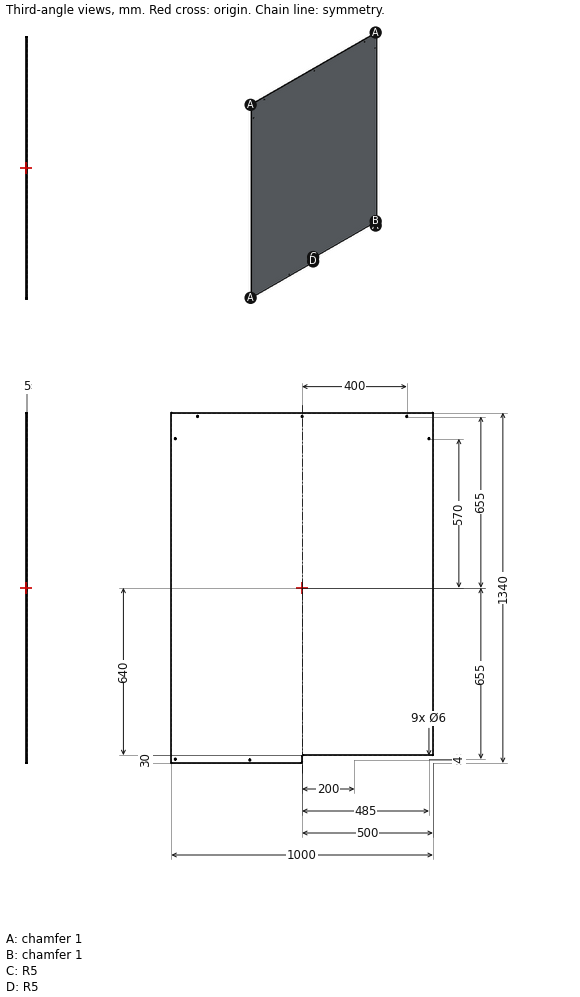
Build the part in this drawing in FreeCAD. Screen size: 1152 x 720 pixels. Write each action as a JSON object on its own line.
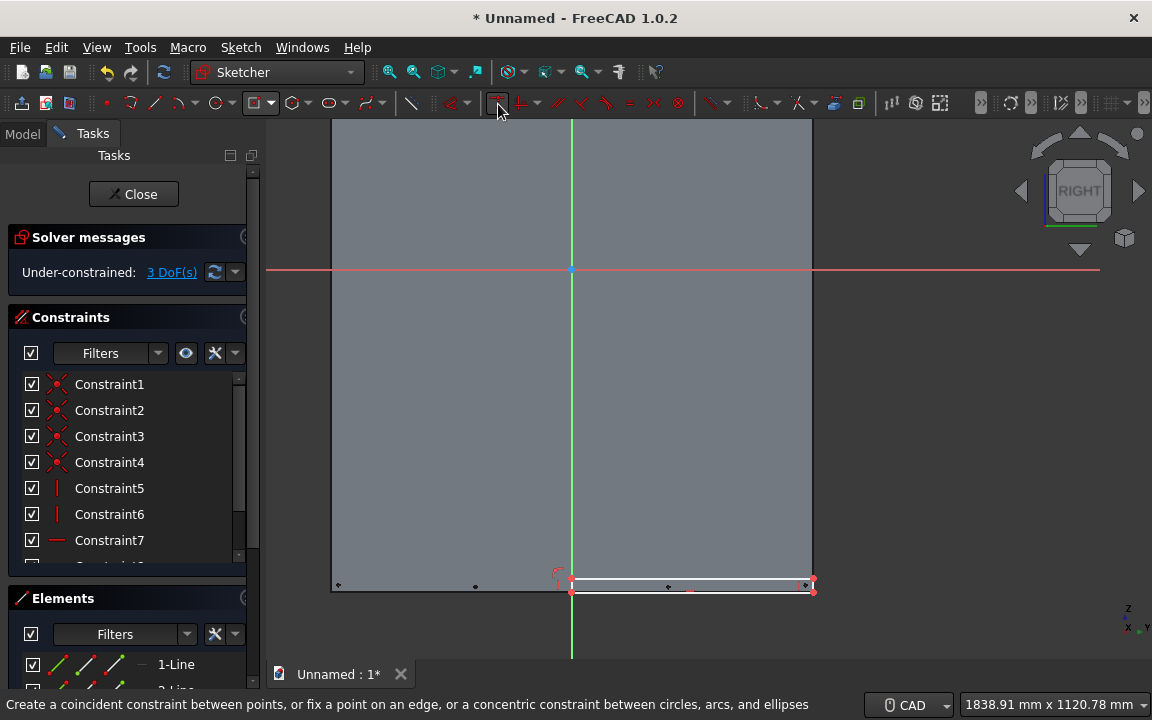
{"action": "left_click", "coordinate": [450, 104]}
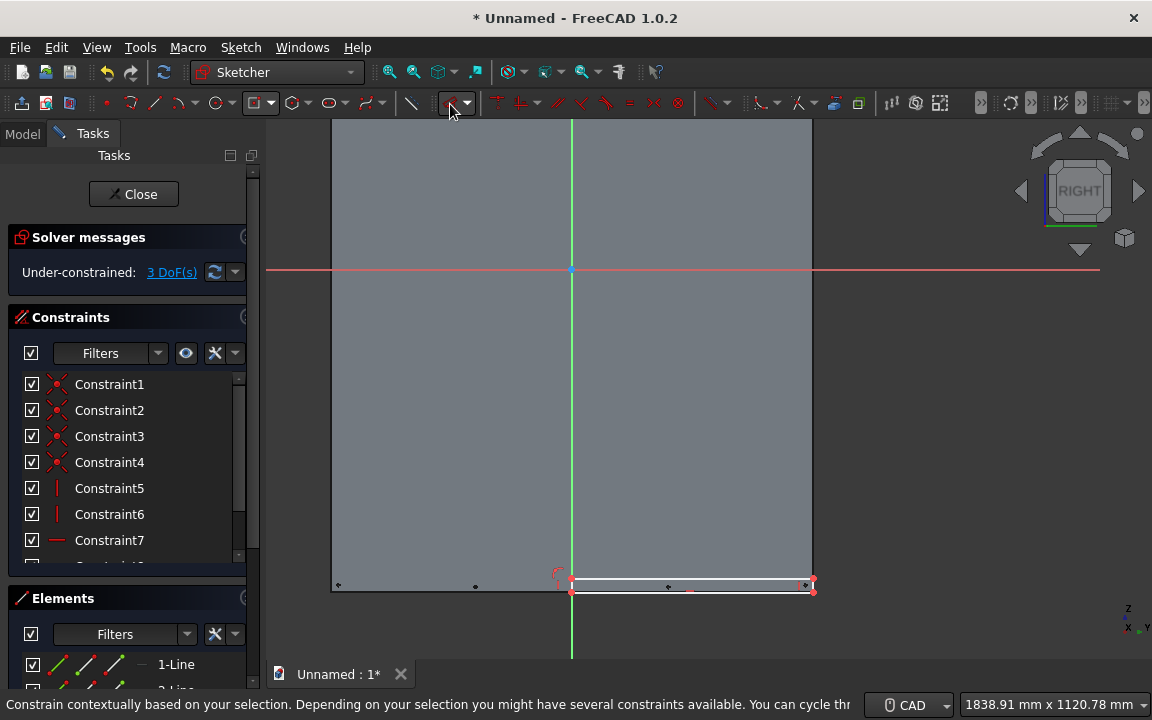
{"action": "scroll", "coordinate": [572, 586], "scroll_direction": "up", "scroll_amount": 6}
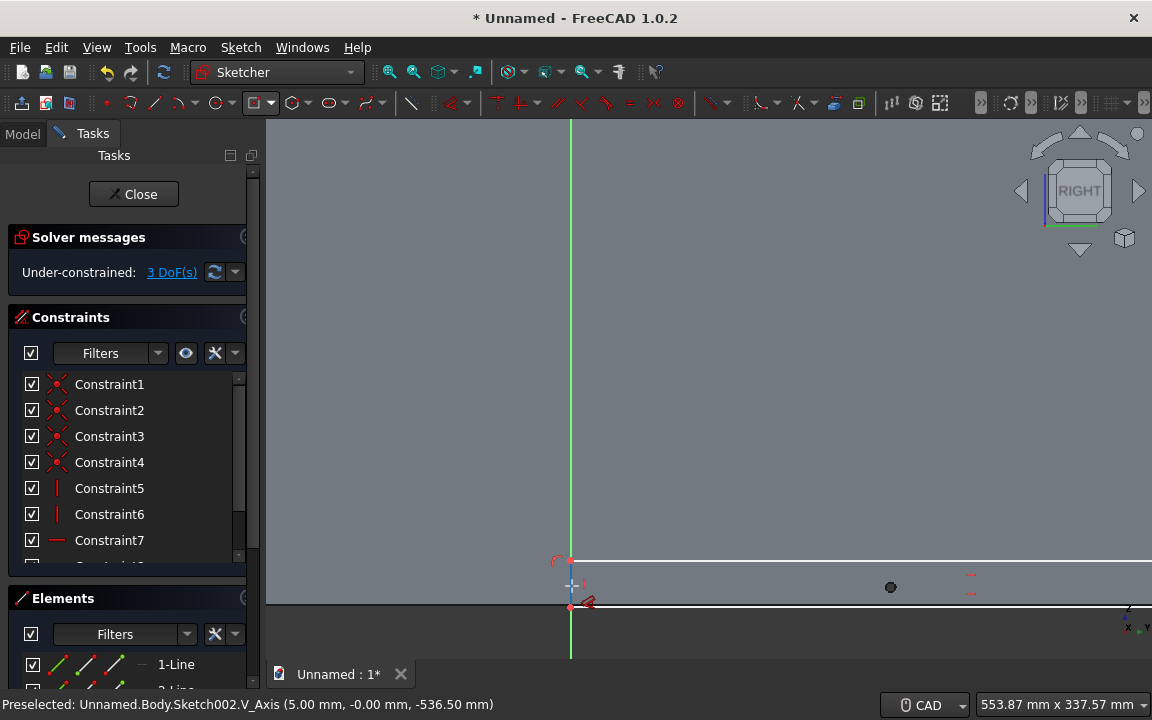
{"action": "left_click", "coordinate": [571, 584]}
{"action": "left_click", "coordinate": [537, 584]}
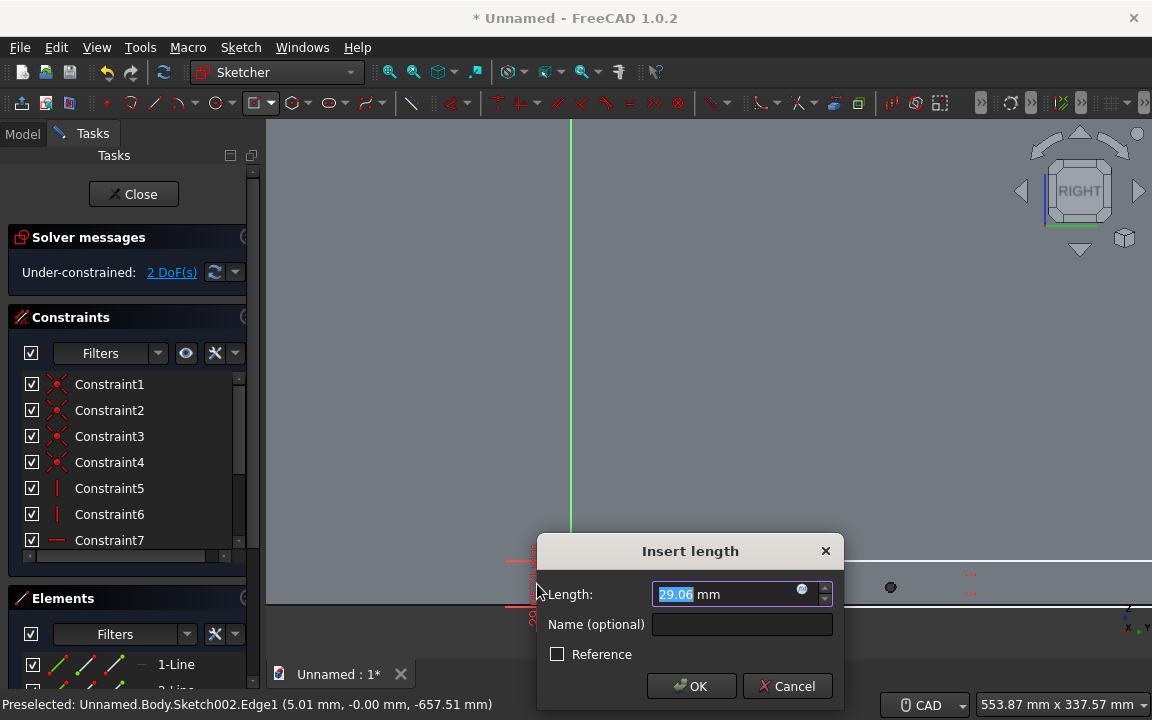
{"action": "type", "text": "30"}
{"action": "key", "text": "Return"}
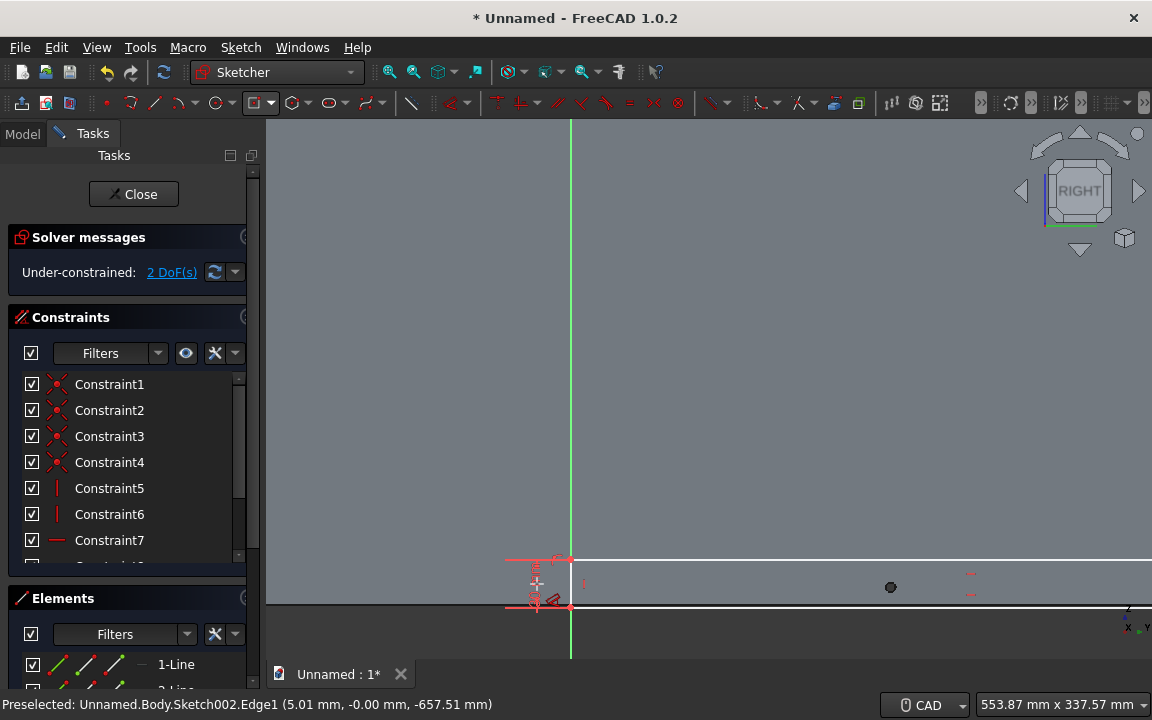
{"action": "left_click", "coordinate": [811, 608]}
{"action": "left_click", "coordinate": [779, 574]}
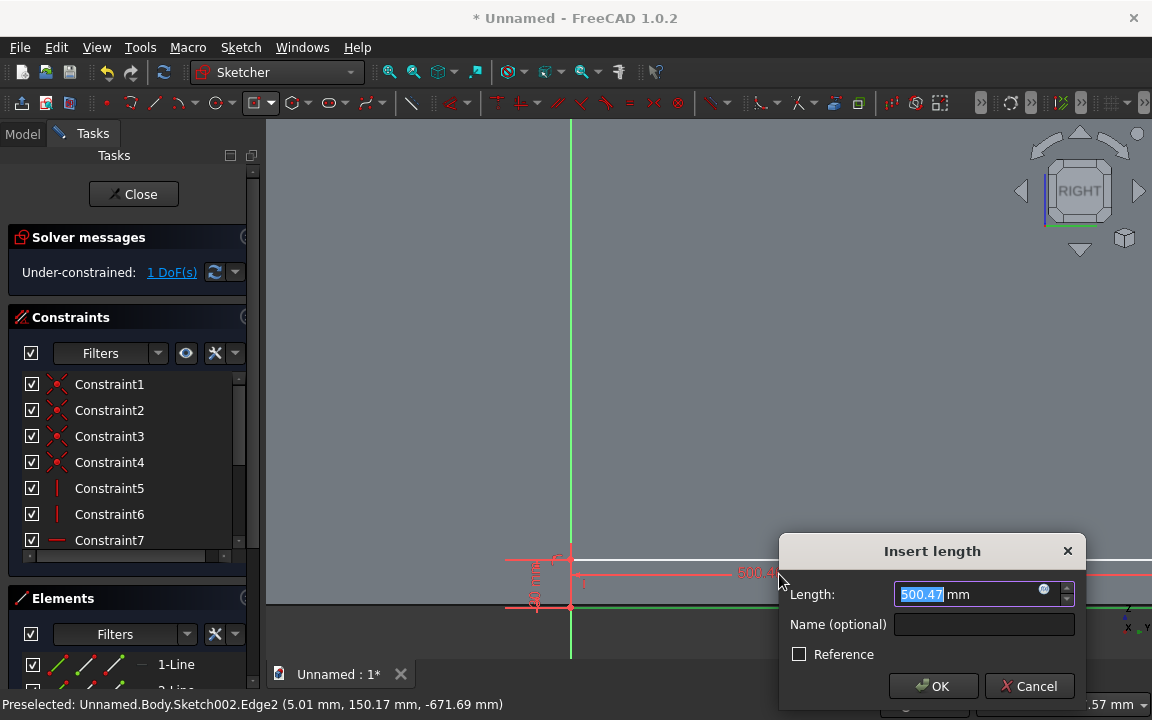
{"action": "type", "text": "500"}
{"action": "key", "text": "Return"}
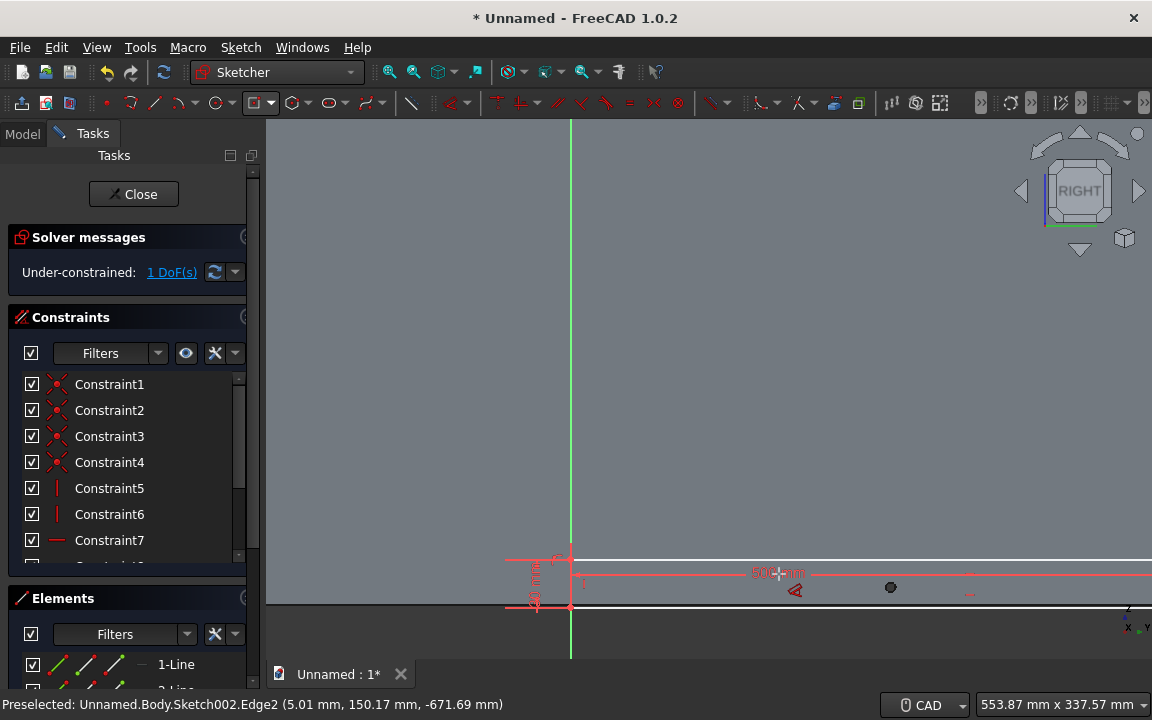
{"action": "left_click", "coordinate": [571, 560]}
{"action": "left_click", "coordinate": [537, 353]}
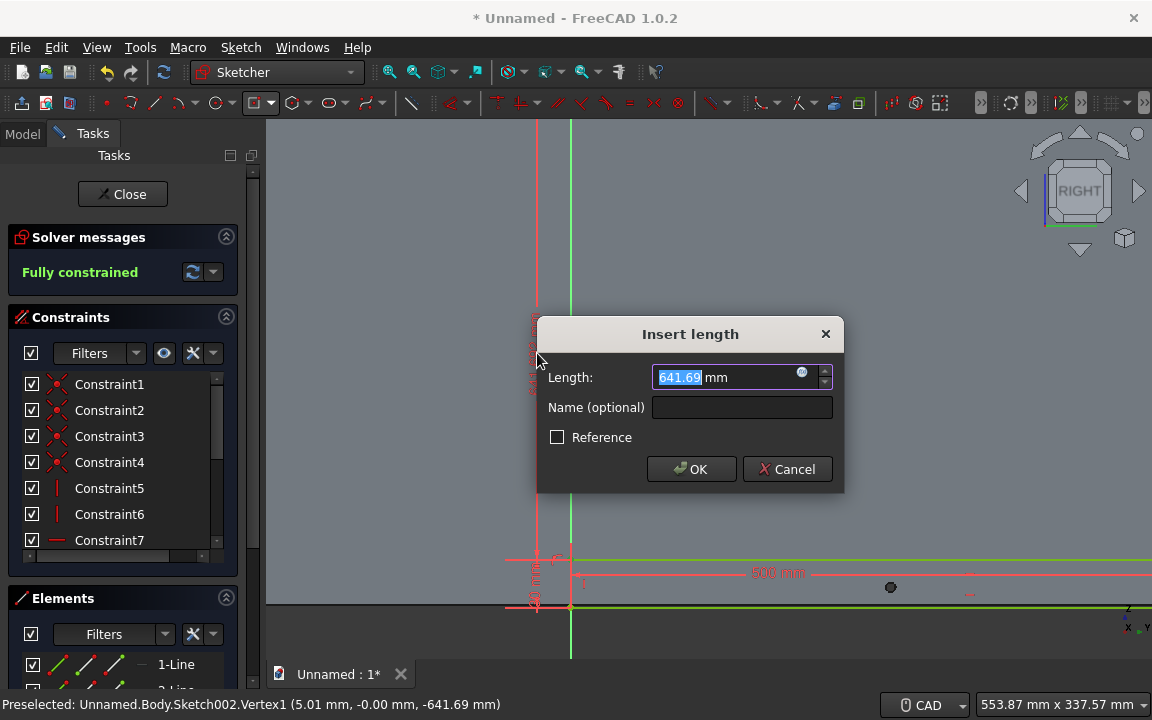
{"action": "type", "text": "640"}
{"action": "key", "text": "Return"}
{"action": "key", "text": "Escape"}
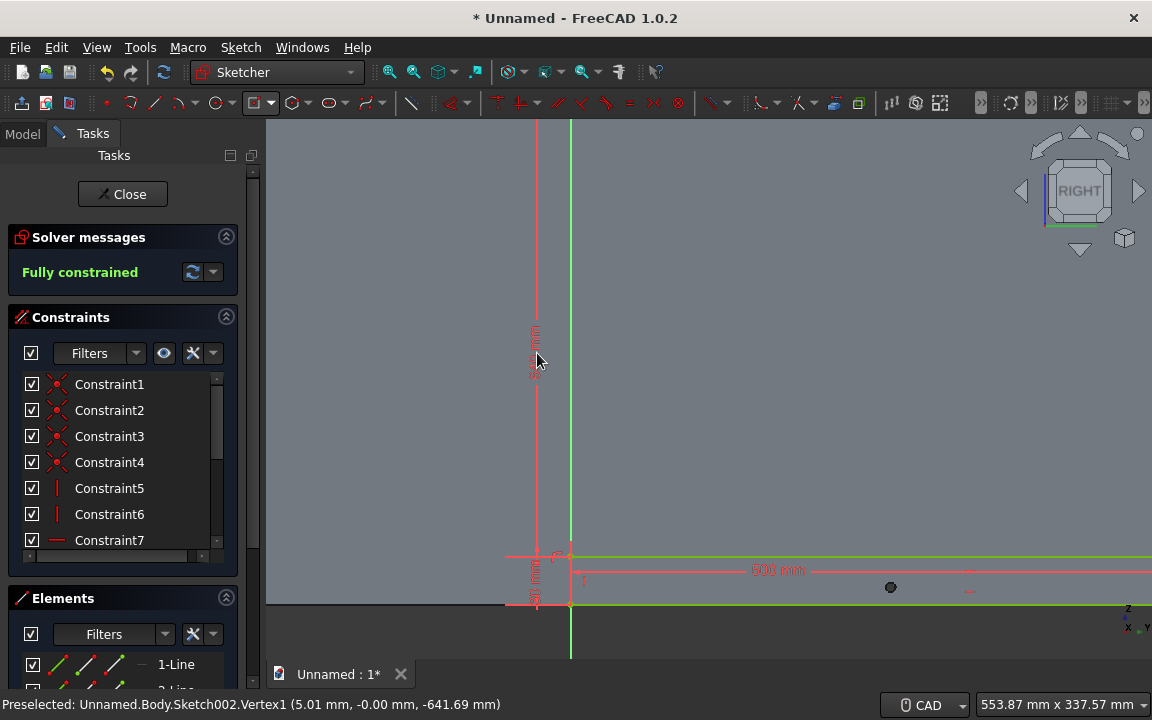
{"action": "left_click", "coordinate": [123, 194]}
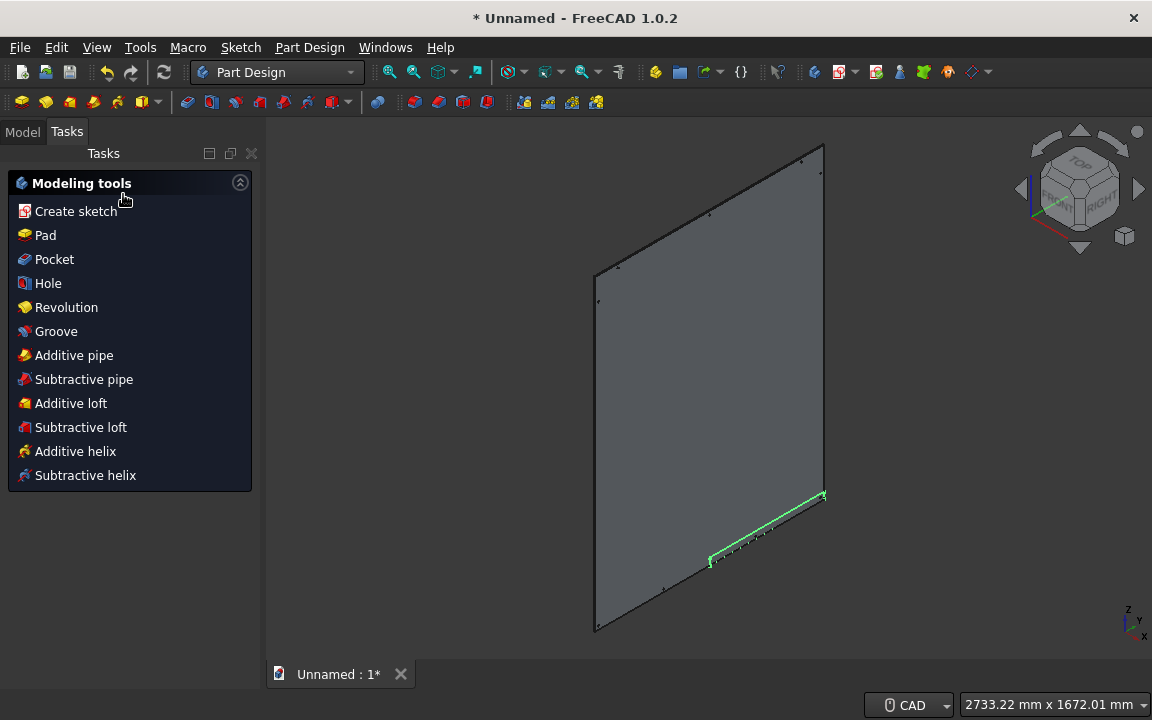
{"action": "left_click", "coordinate": [188, 102]}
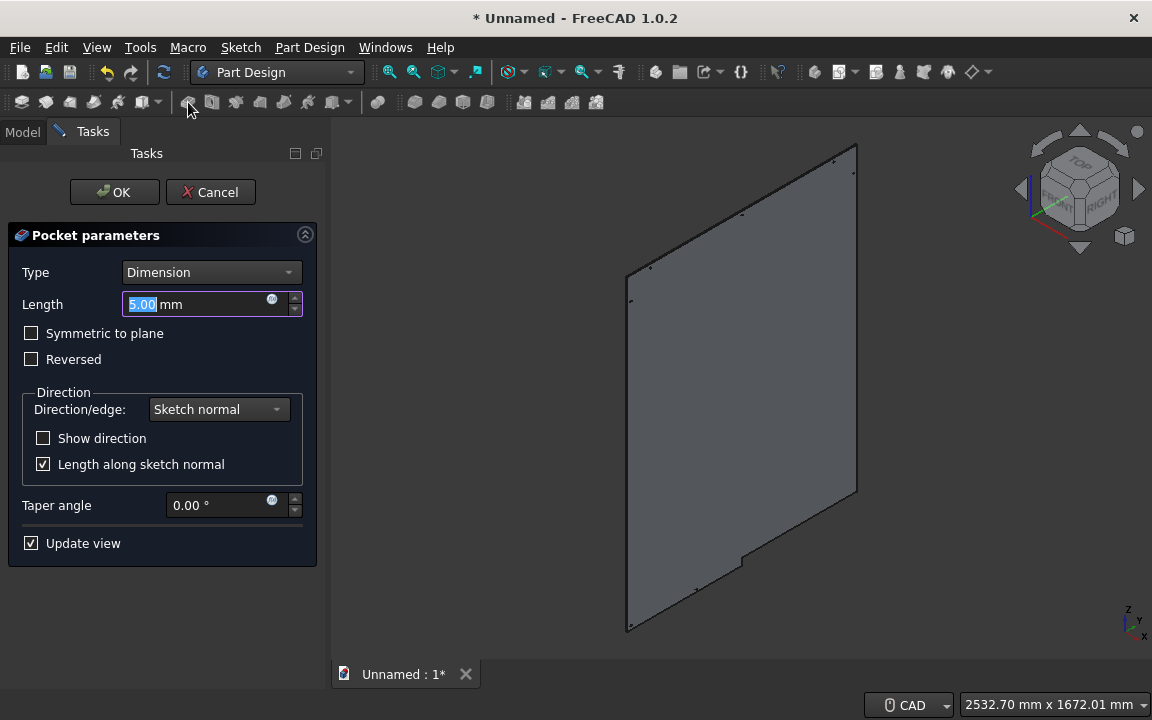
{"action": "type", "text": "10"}
{"action": "key", "text": "Tab"}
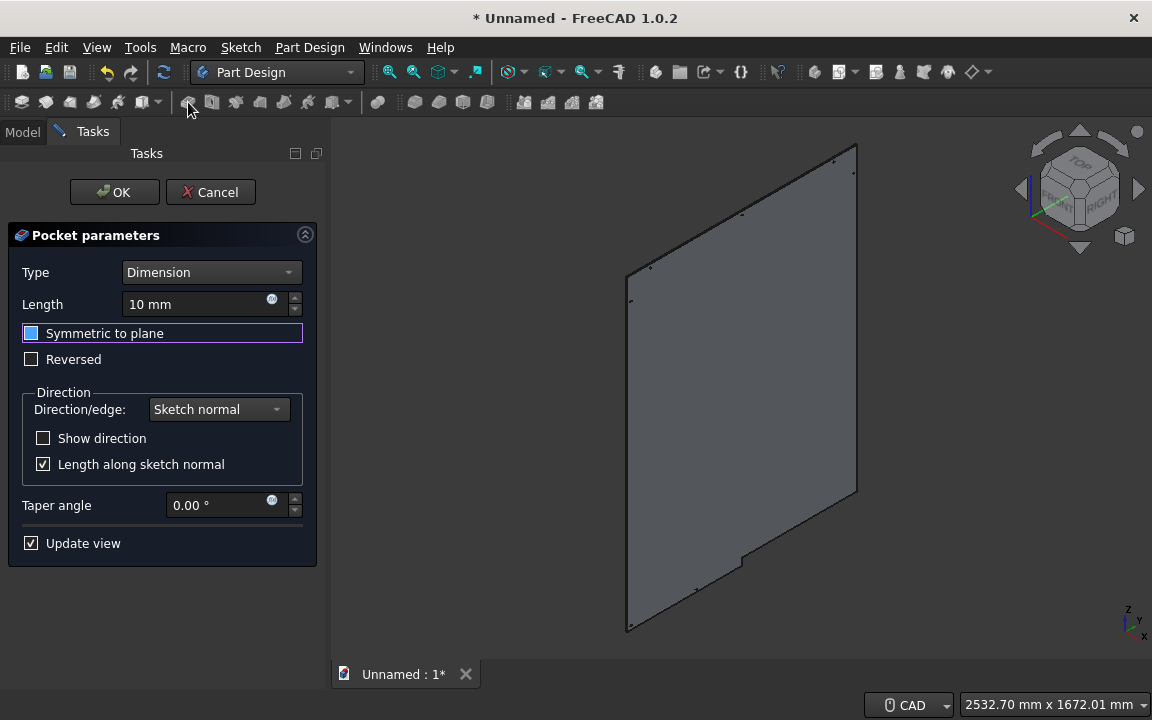
{"action": "left_click", "coordinate": [115, 192]}